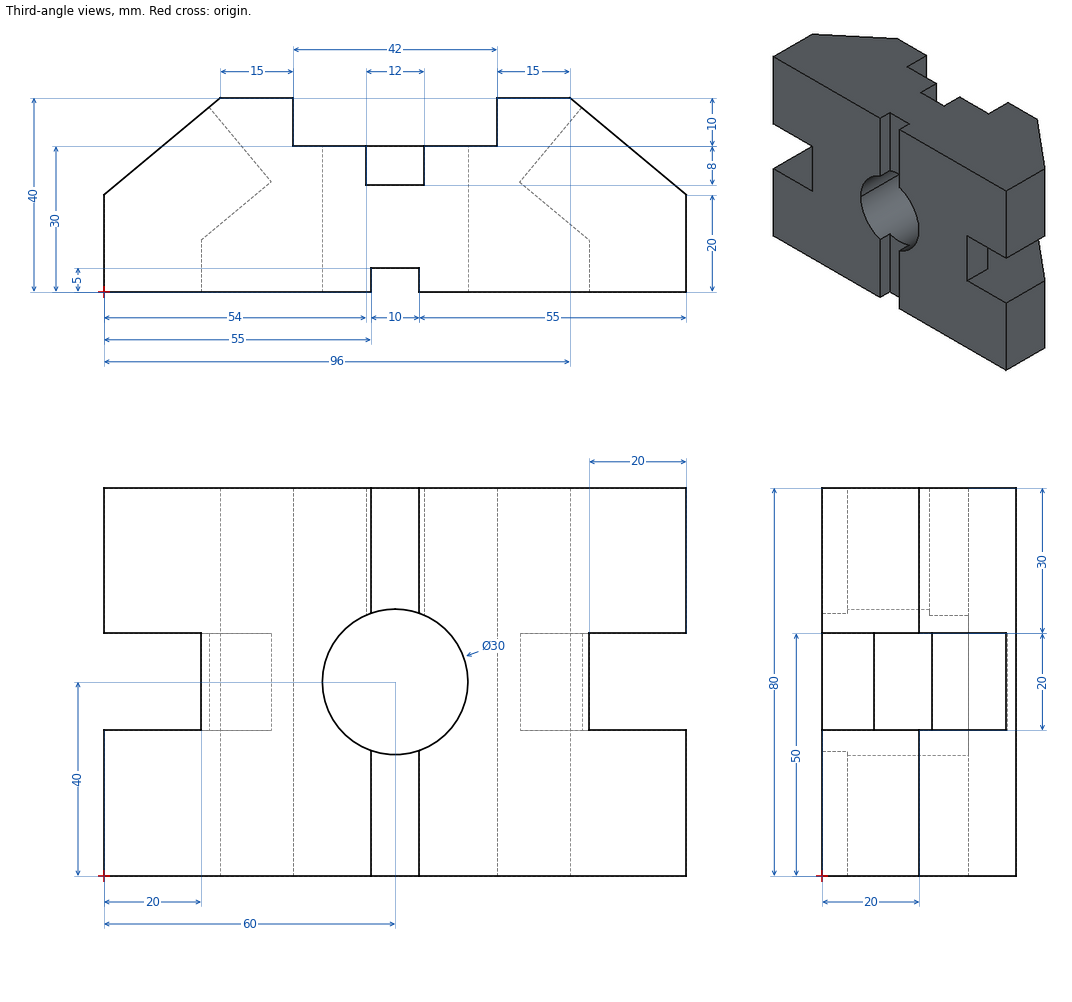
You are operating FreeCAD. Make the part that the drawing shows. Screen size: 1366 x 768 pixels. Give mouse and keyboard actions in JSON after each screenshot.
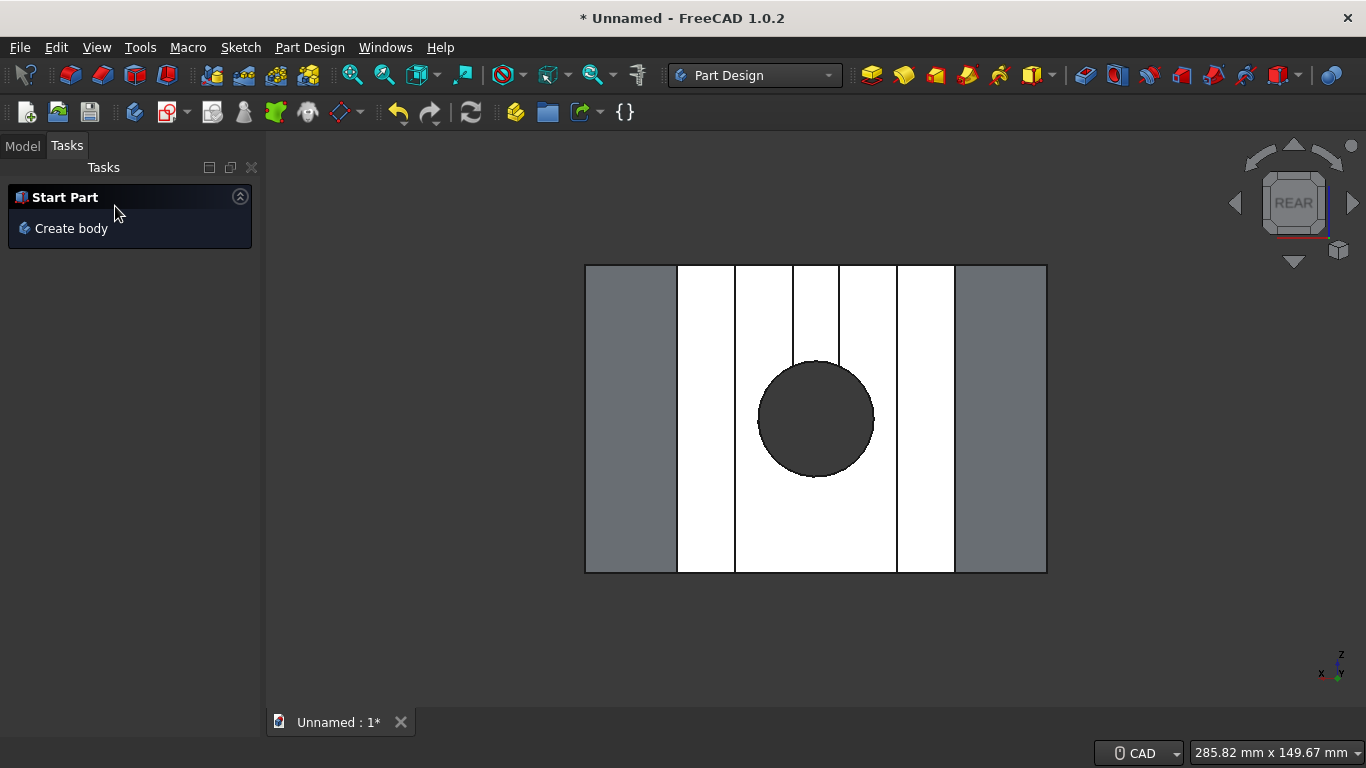
{"action": "left_click", "coordinate": [631, 330]}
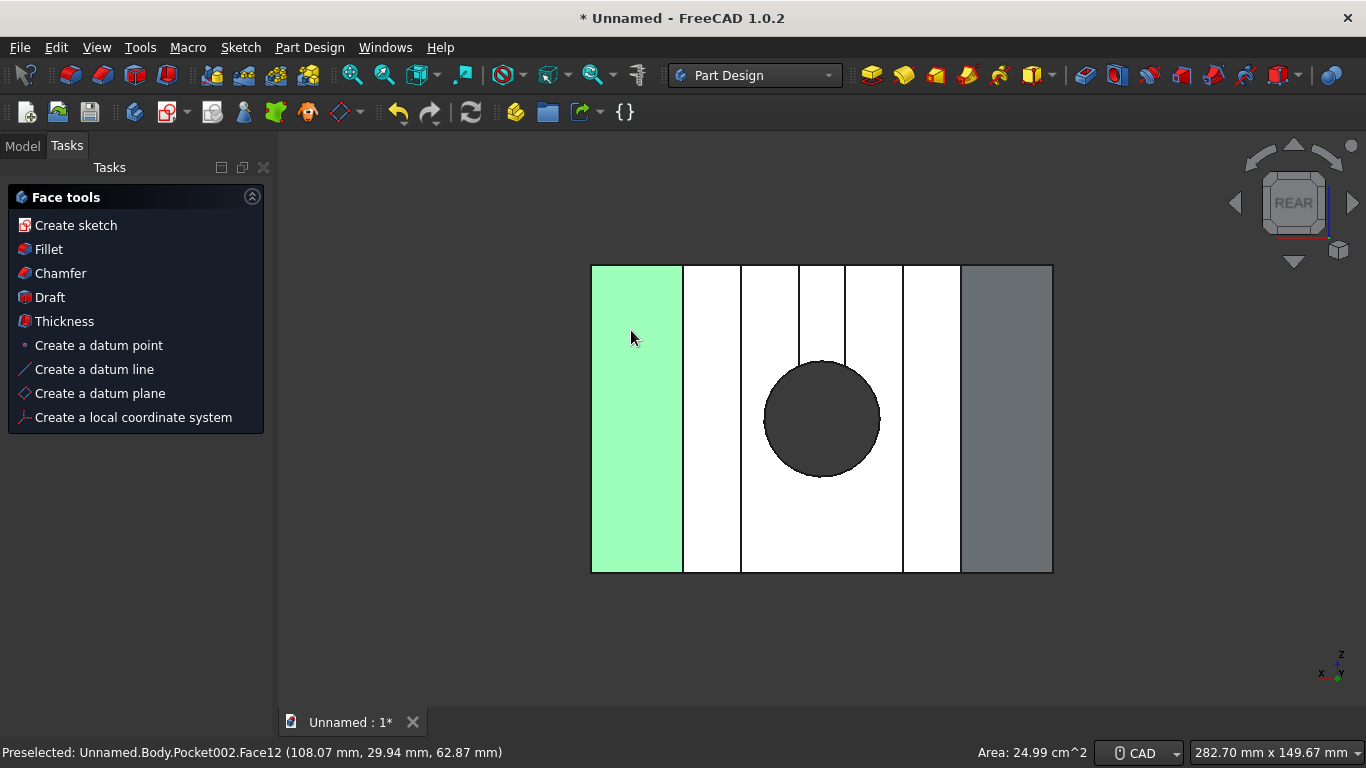
{"action": "left_click", "coordinate": [168, 112]}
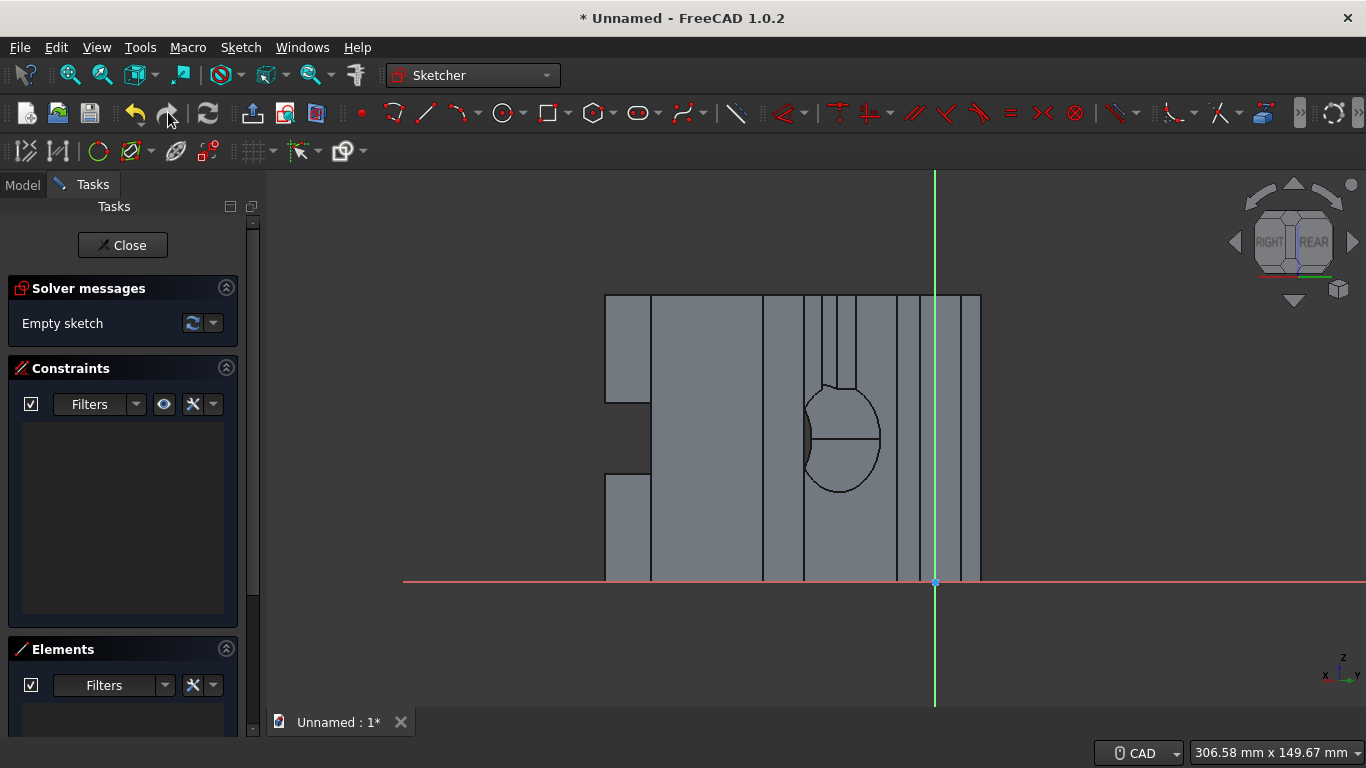
{"action": "scroll", "coordinate": [689, 438], "scroll_direction": "up", "scroll_amount": 8}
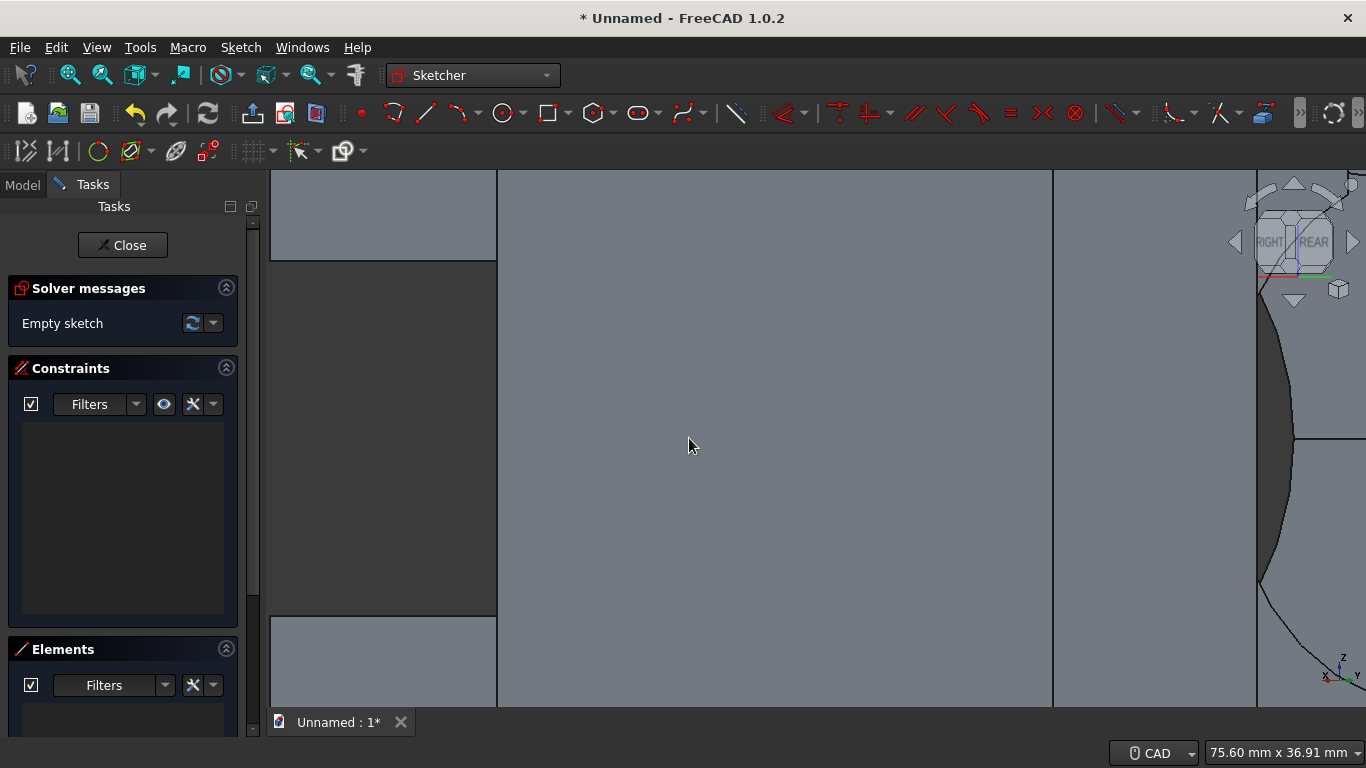
{"action": "key", "text": "g r"}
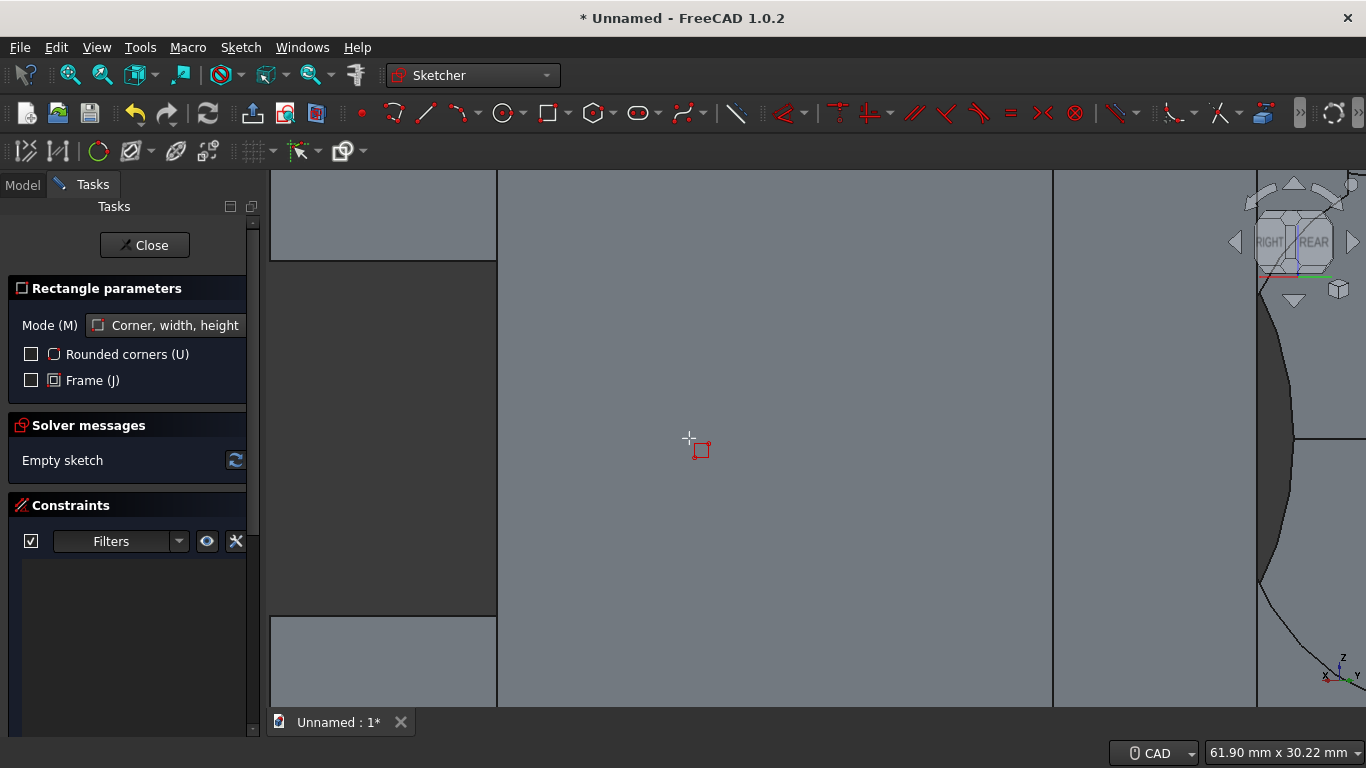
{"action": "left_click", "coordinate": [497, 261]}
{"action": "mouse_move", "coordinate": [996, 616]}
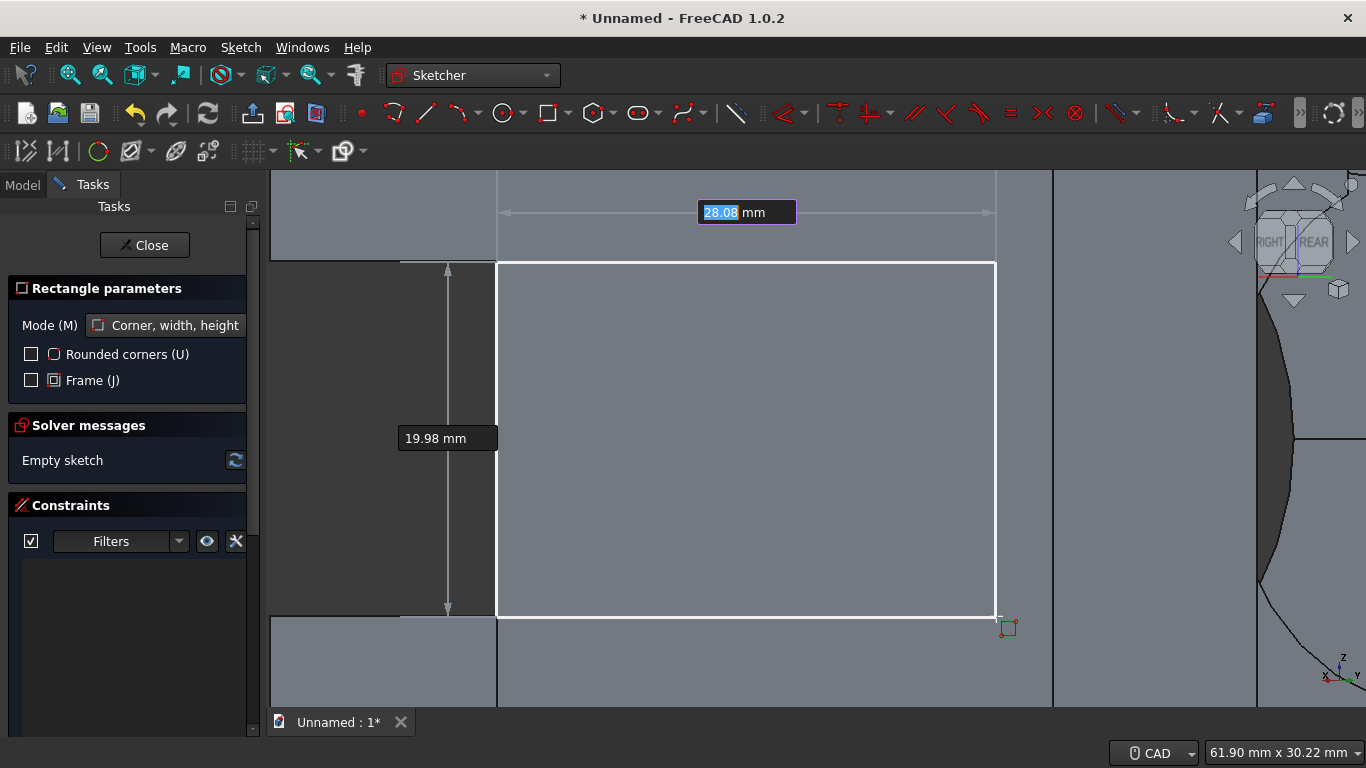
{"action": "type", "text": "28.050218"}
{"action": "key", "text": "Tab"}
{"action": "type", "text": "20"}
{"action": "key", "text": "Return"}
{"action": "key", "text": "Escape"}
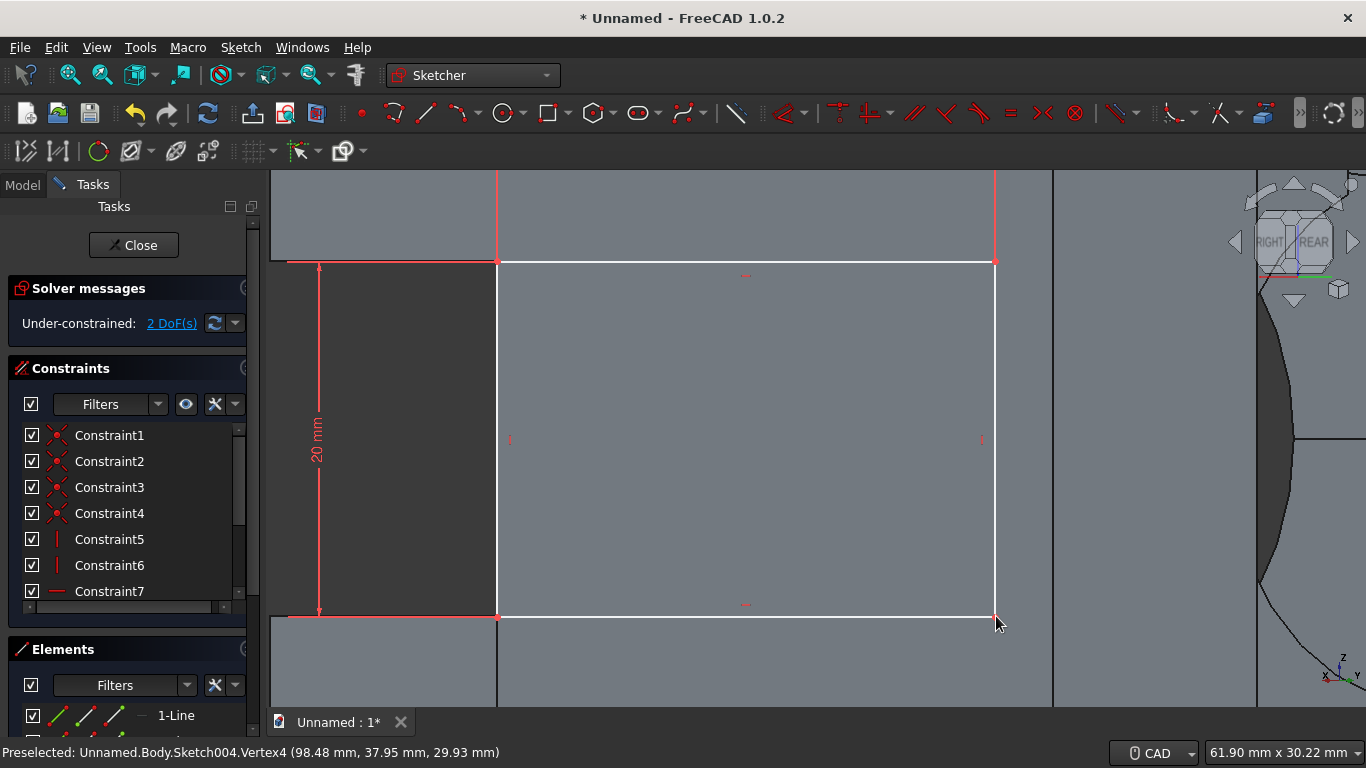
{"action": "key", "text": "d"}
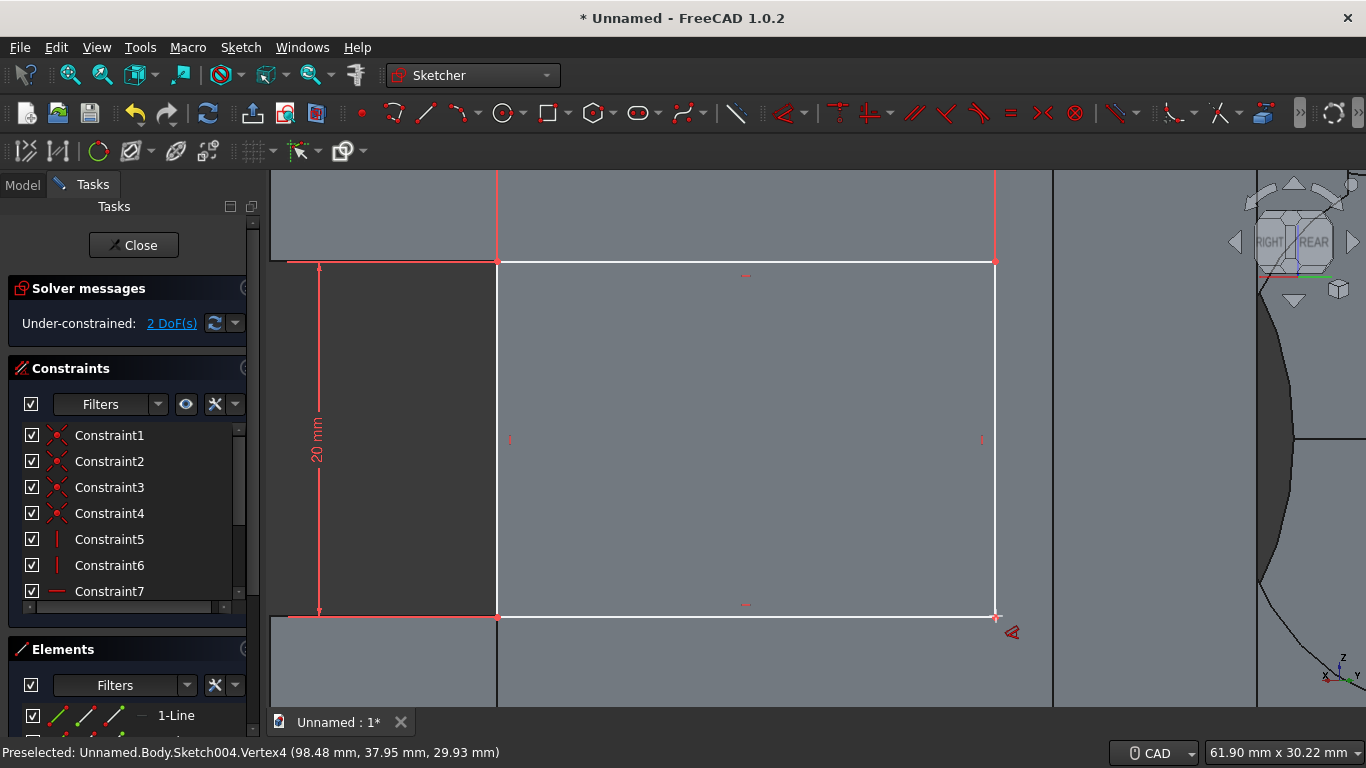
{"action": "left_click", "coordinate": [497, 262]}
{"action": "left_click", "coordinate": [463, 471]}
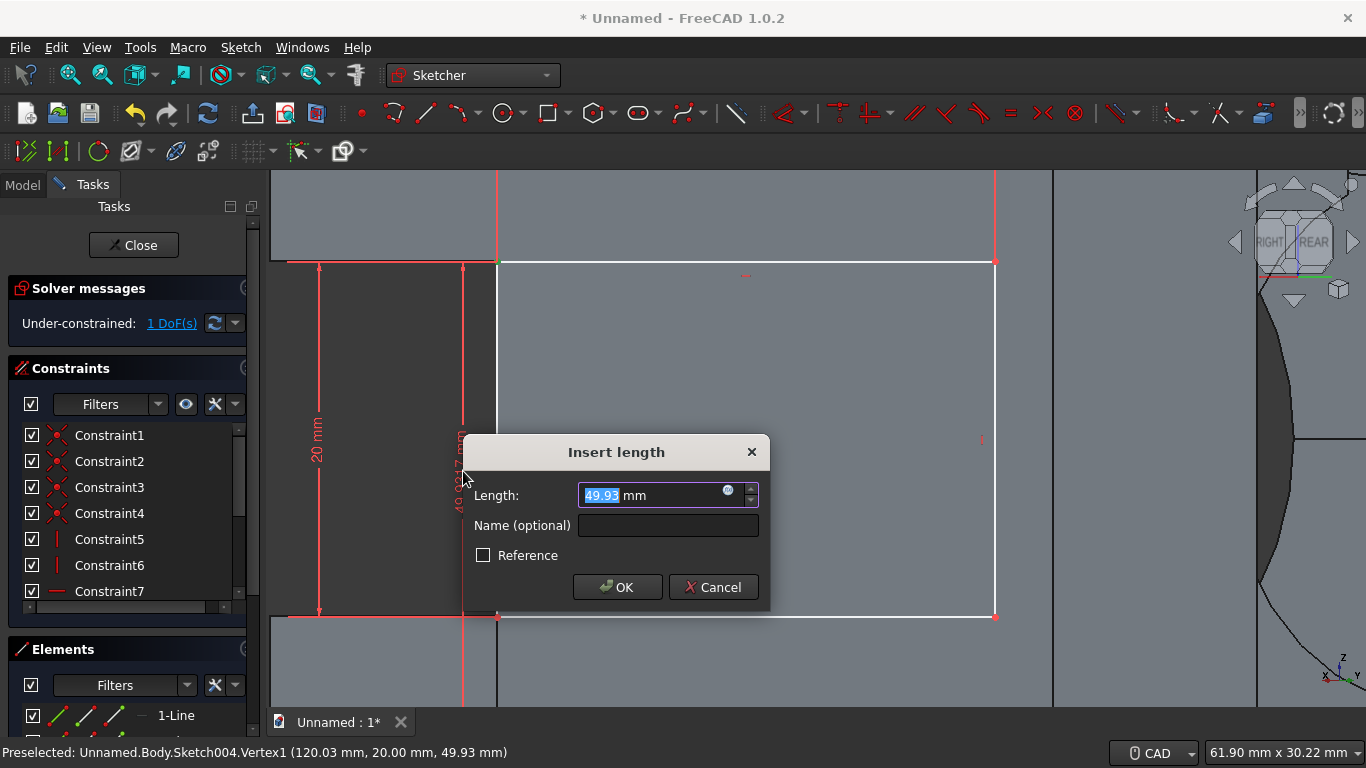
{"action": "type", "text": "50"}
{"action": "key", "text": "Return"}